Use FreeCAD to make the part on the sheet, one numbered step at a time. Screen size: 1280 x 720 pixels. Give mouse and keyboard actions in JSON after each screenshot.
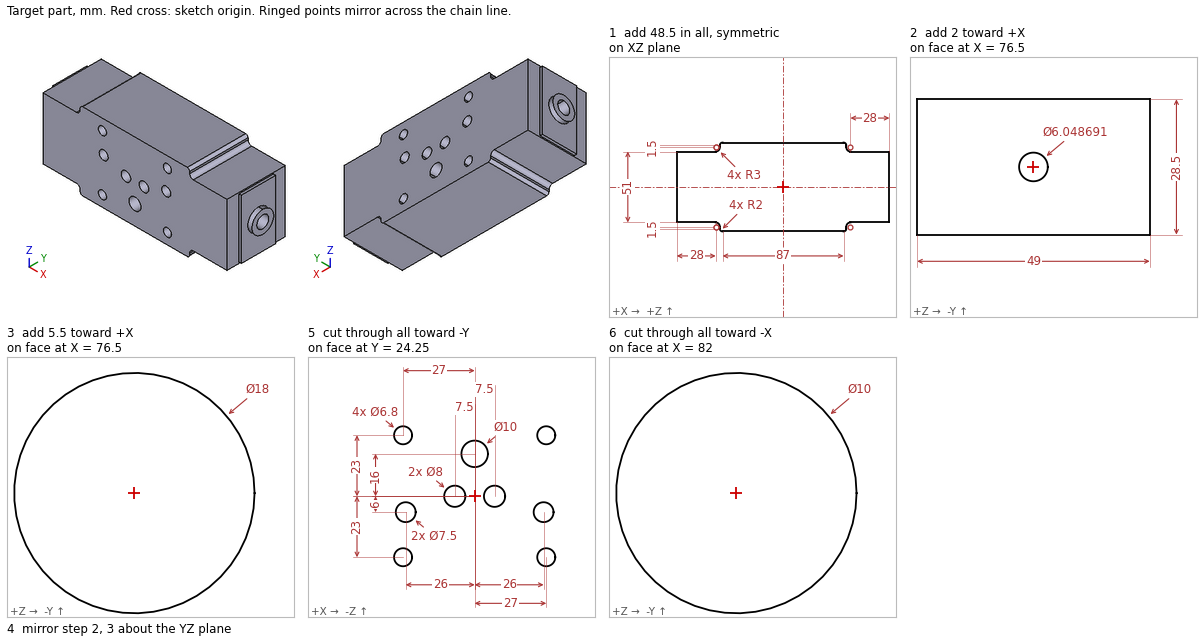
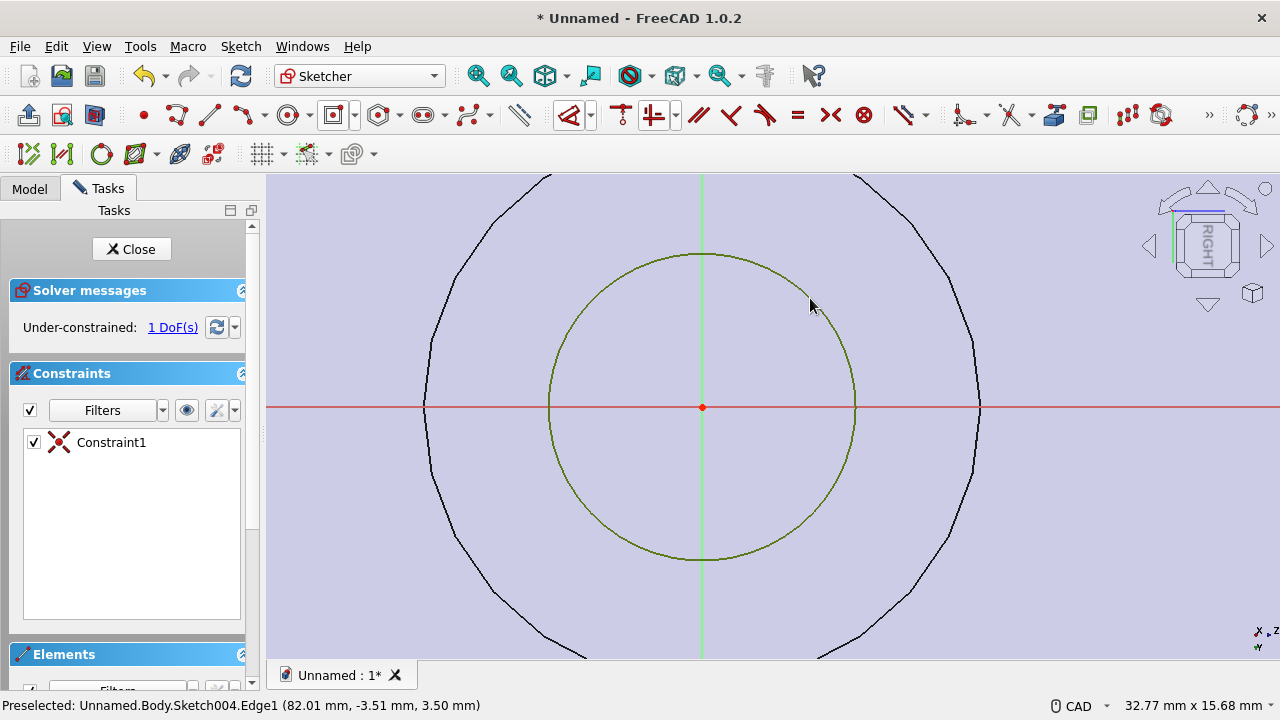
{"action": "left_click", "coordinate": [590, 116]}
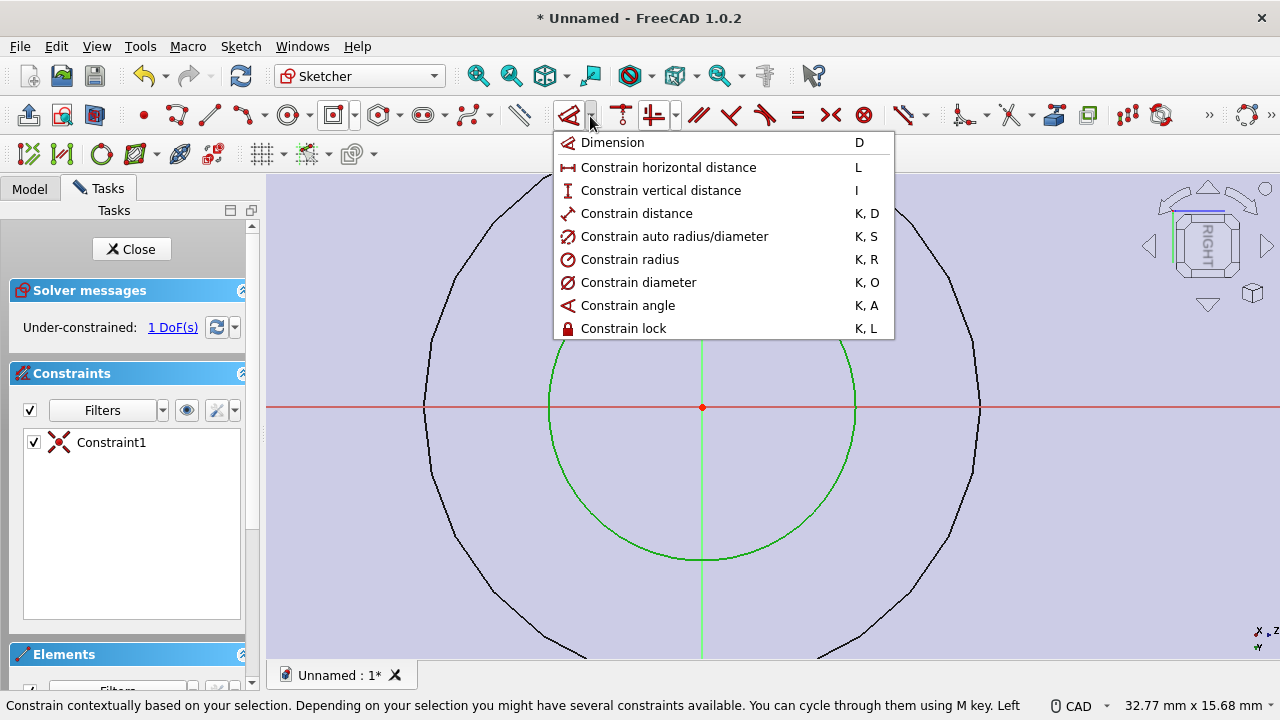
{"action": "left_click", "coordinate": [724, 282]}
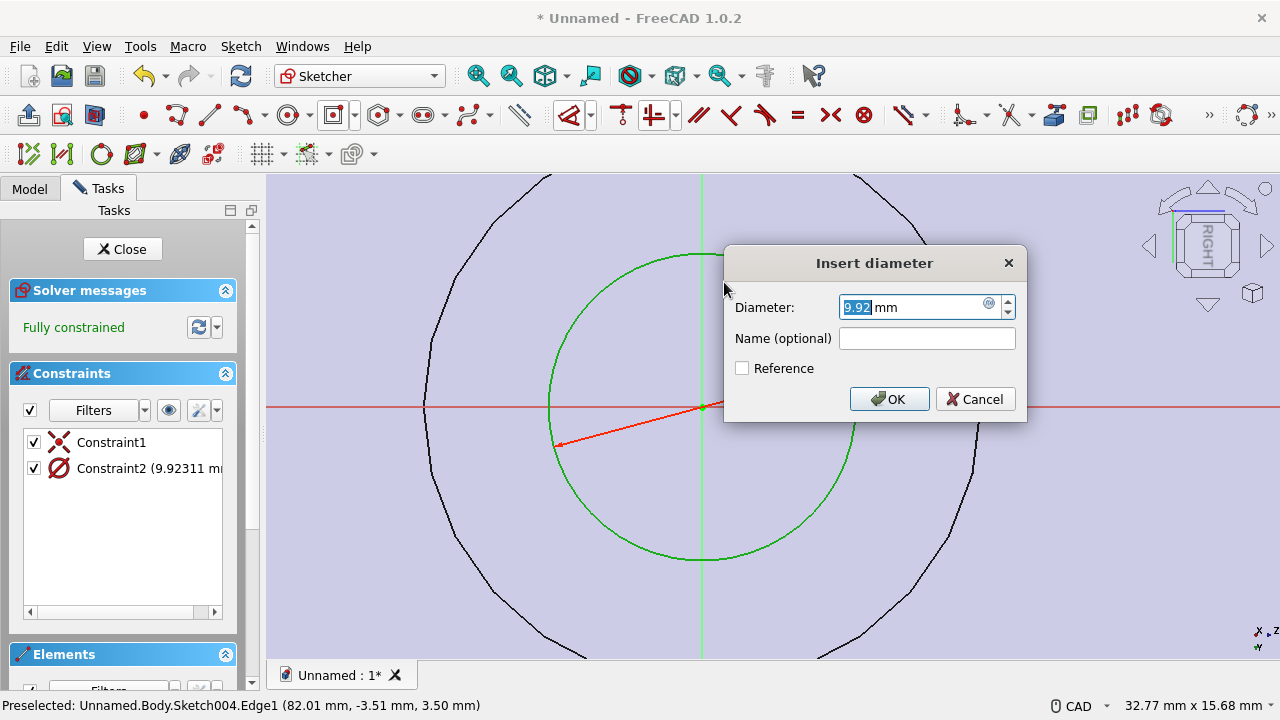
{"action": "type", "text": "10"}
{"action": "key", "text": "Return"}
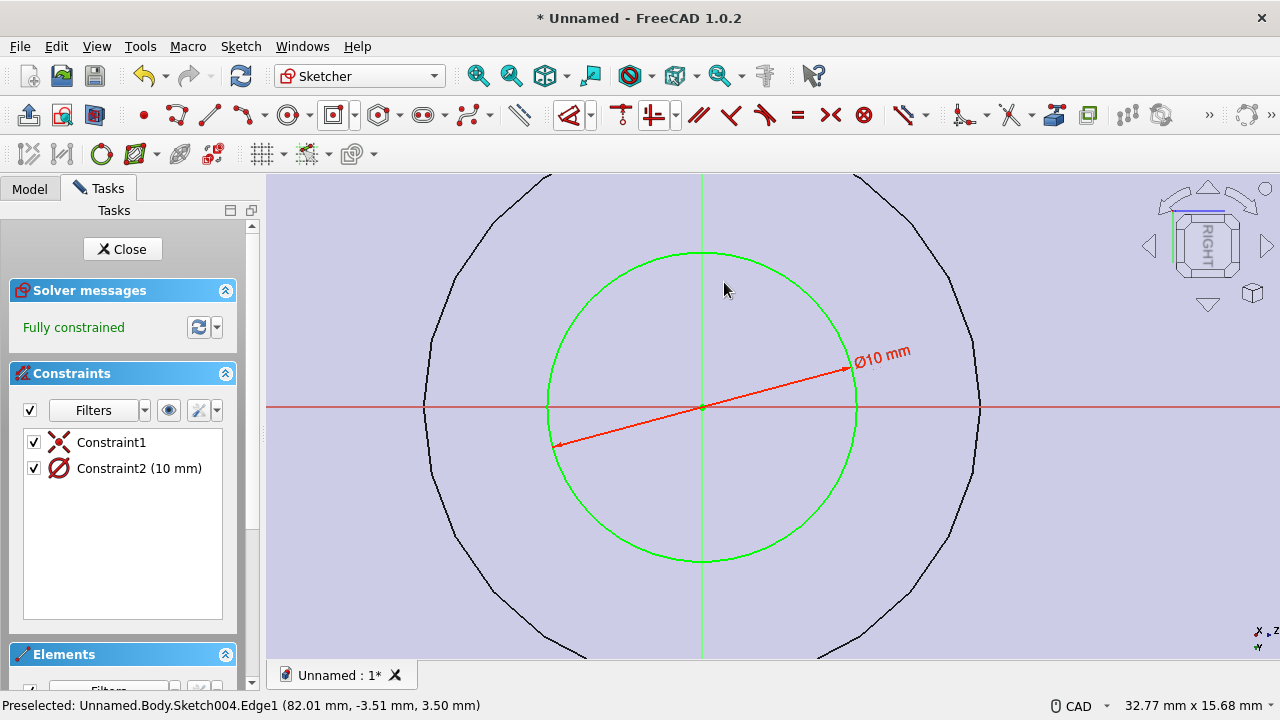
{"action": "left_click", "coordinate": [123, 249]}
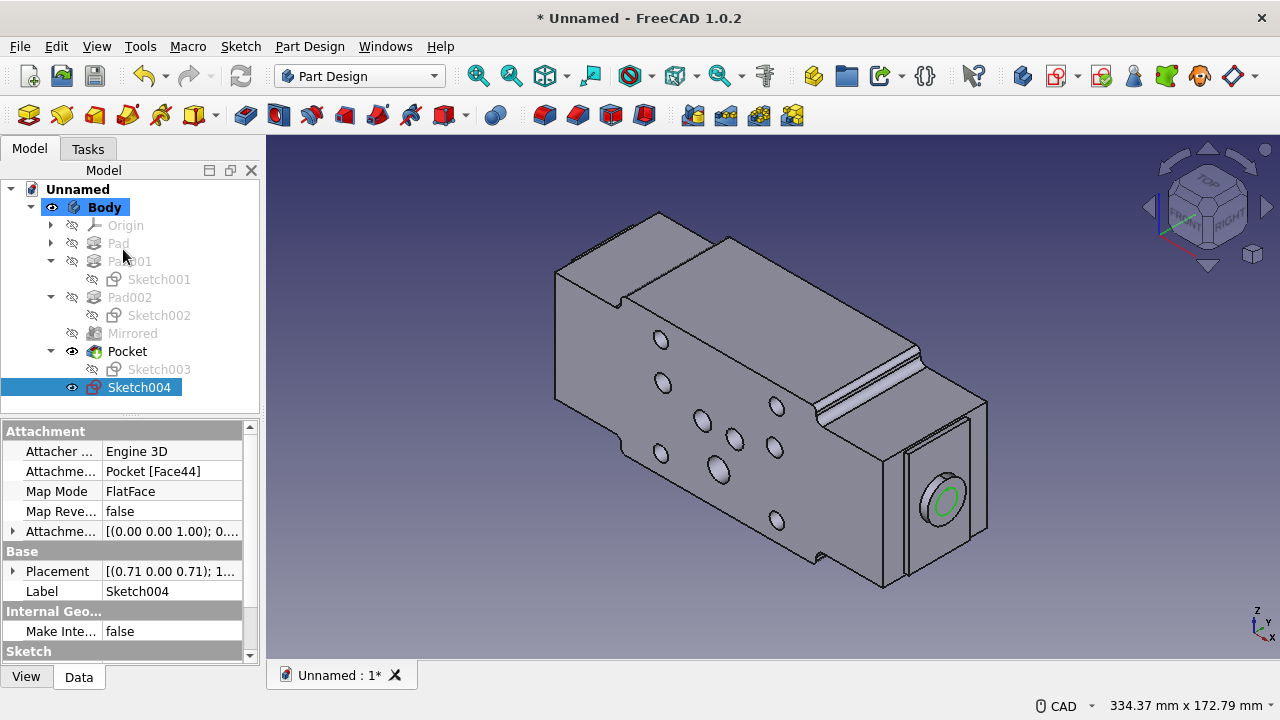
{"action": "left_click", "coordinate": [246, 116]}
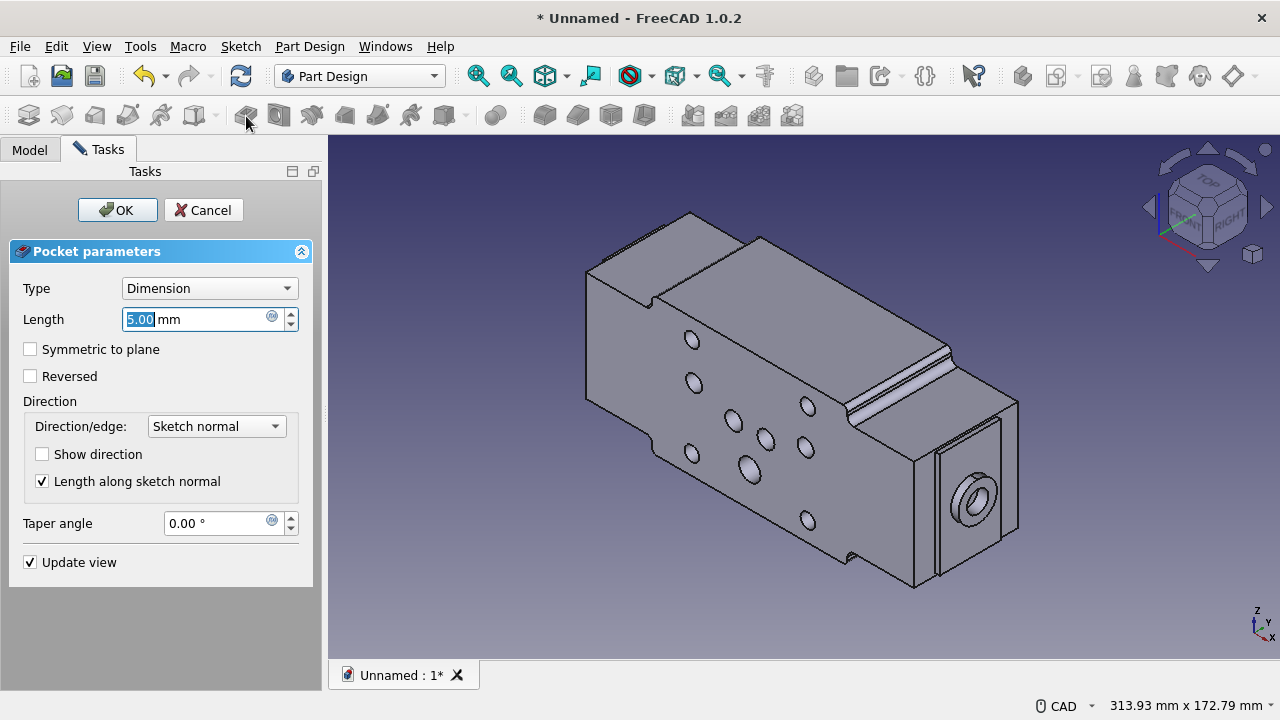
{"action": "left_click", "coordinate": [210, 288]}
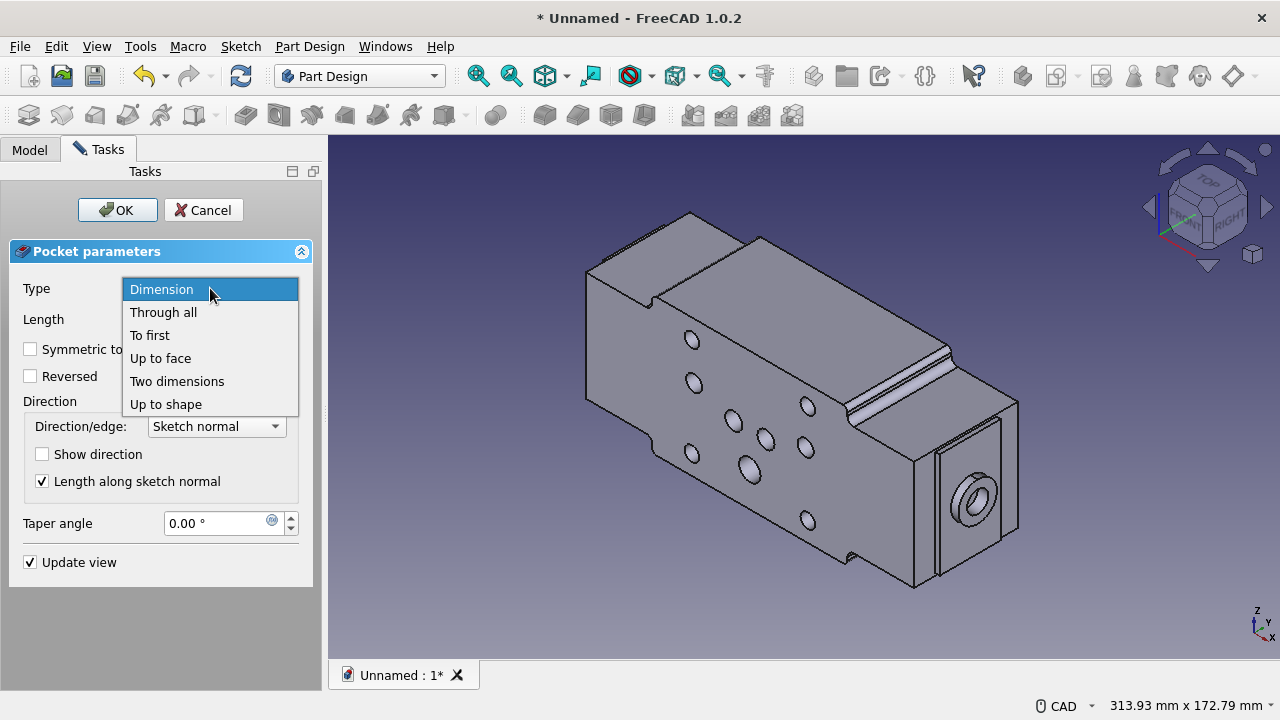
{"action": "left_click", "coordinate": [208, 312]}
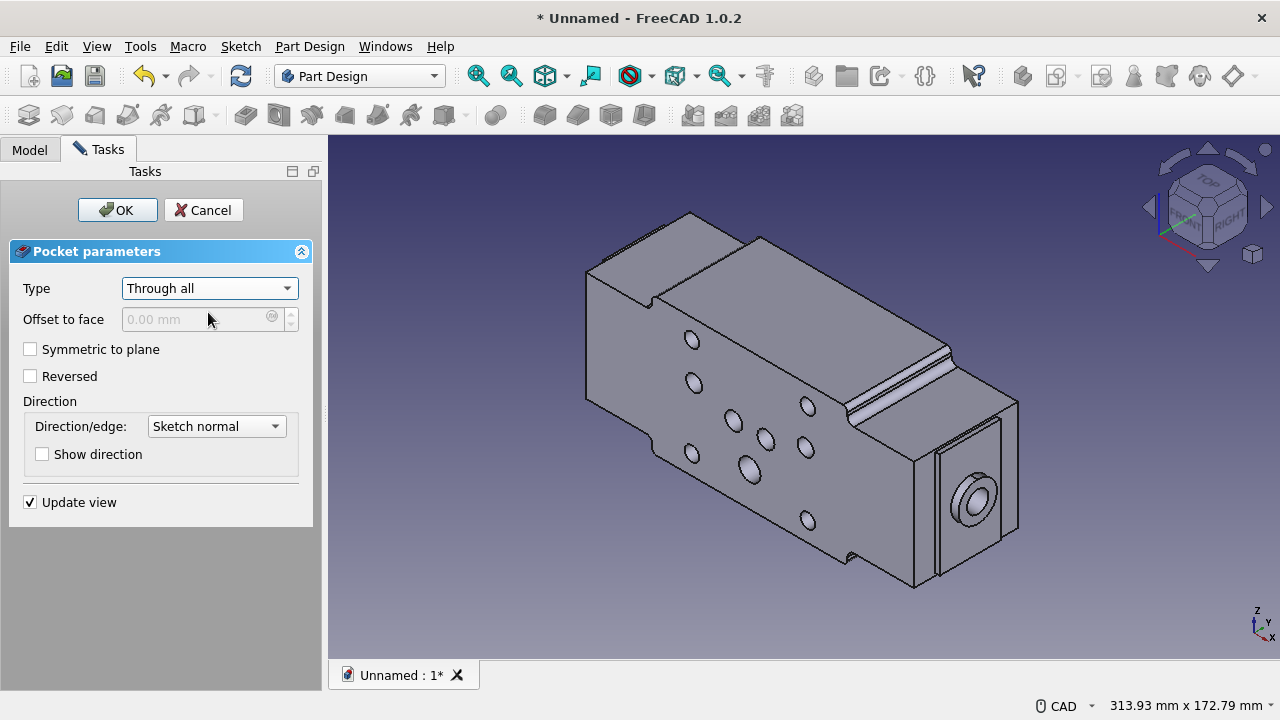
{"action": "left_click", "coordinate": [118, 210]}